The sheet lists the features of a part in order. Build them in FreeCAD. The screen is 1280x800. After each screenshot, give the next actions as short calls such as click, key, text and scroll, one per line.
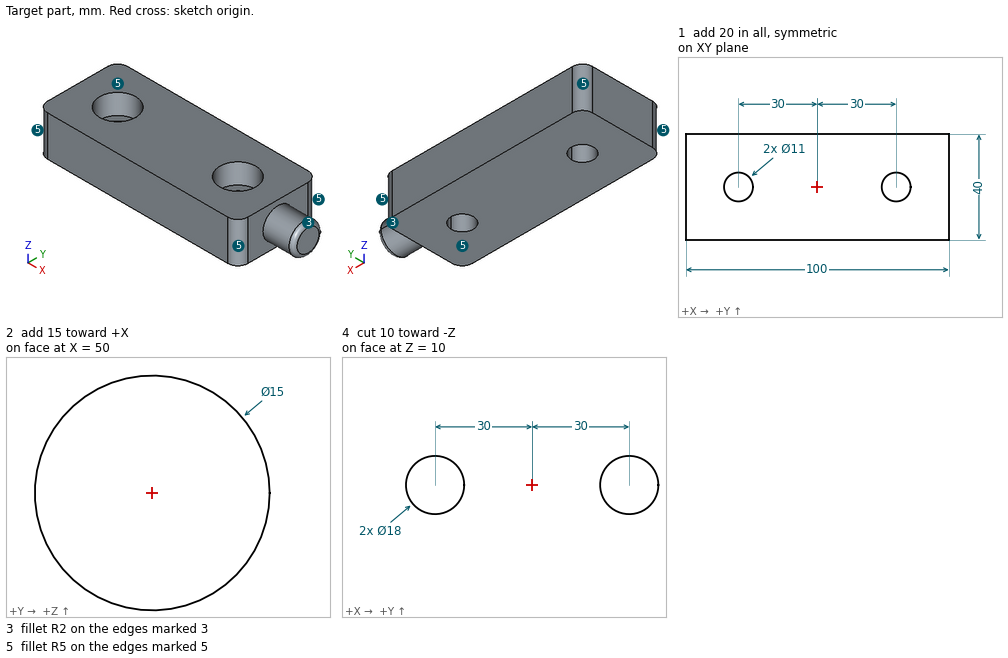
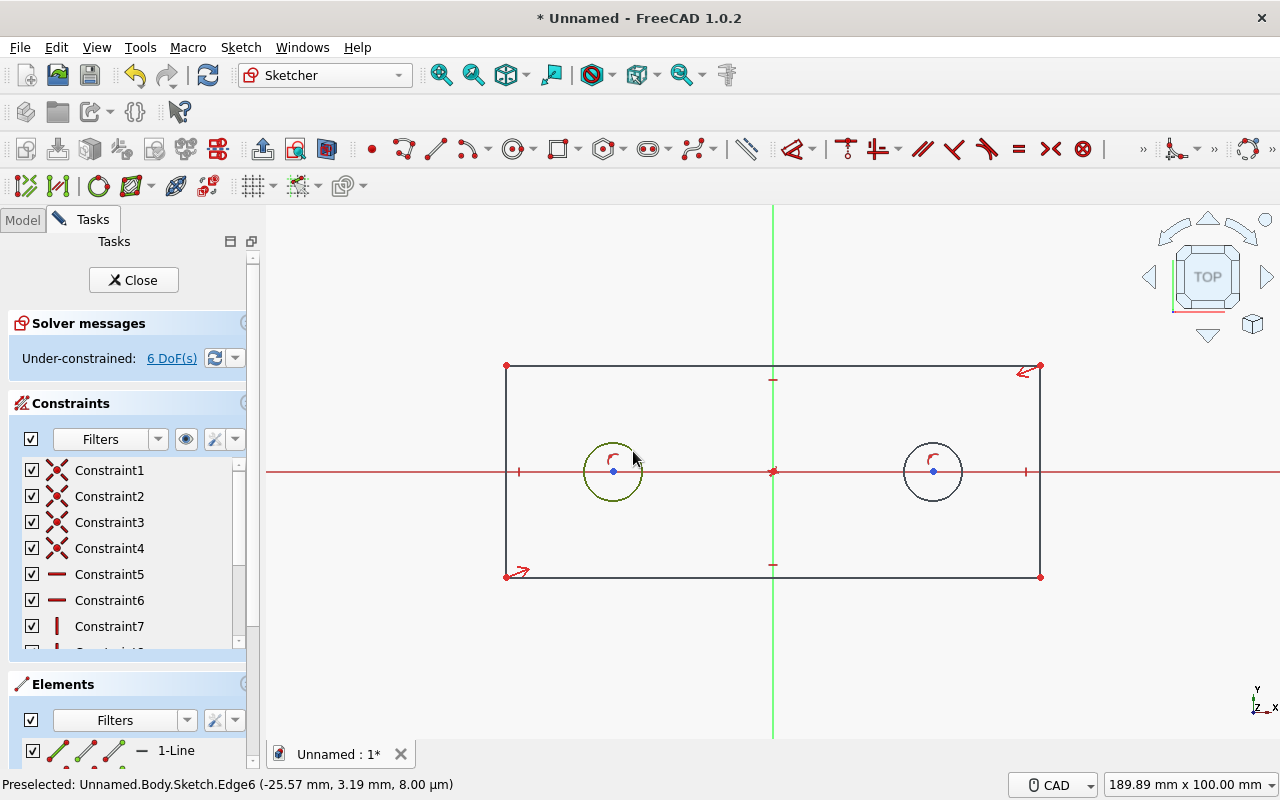
click(953, 451)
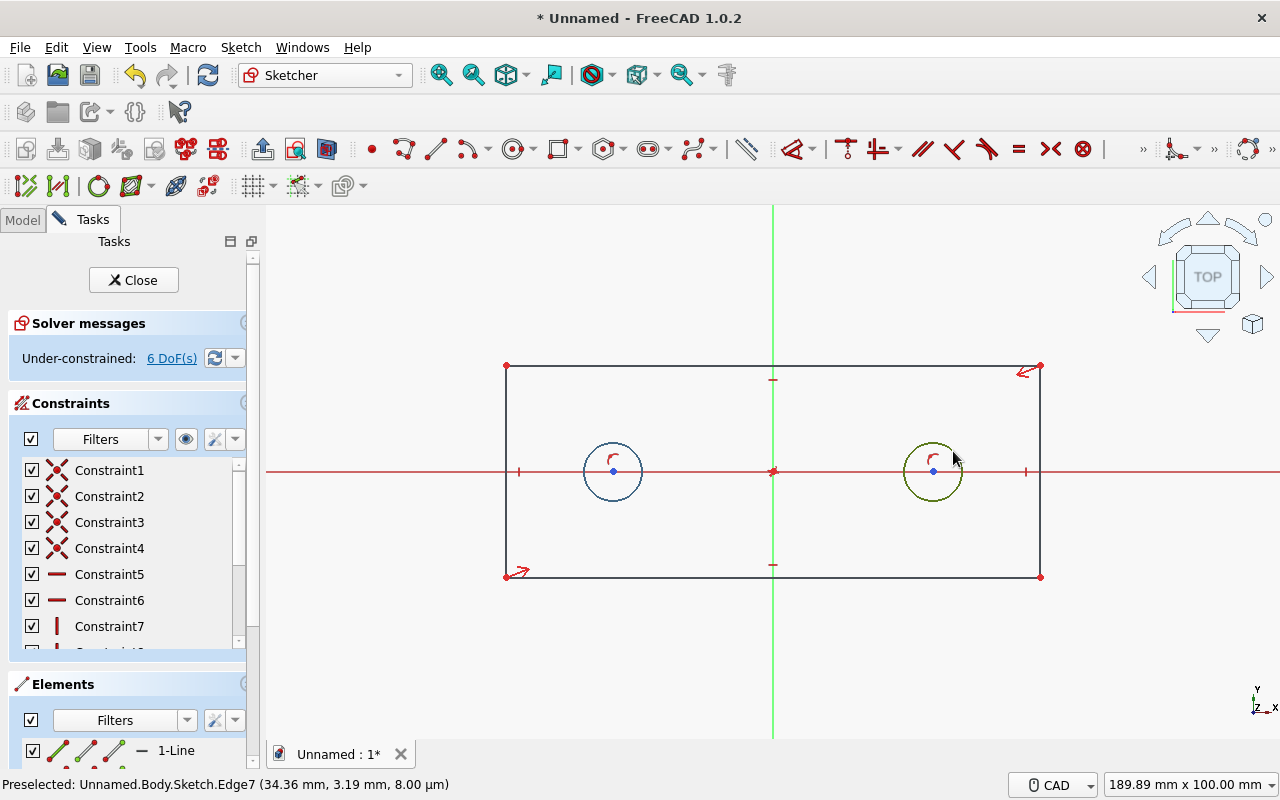
key(e)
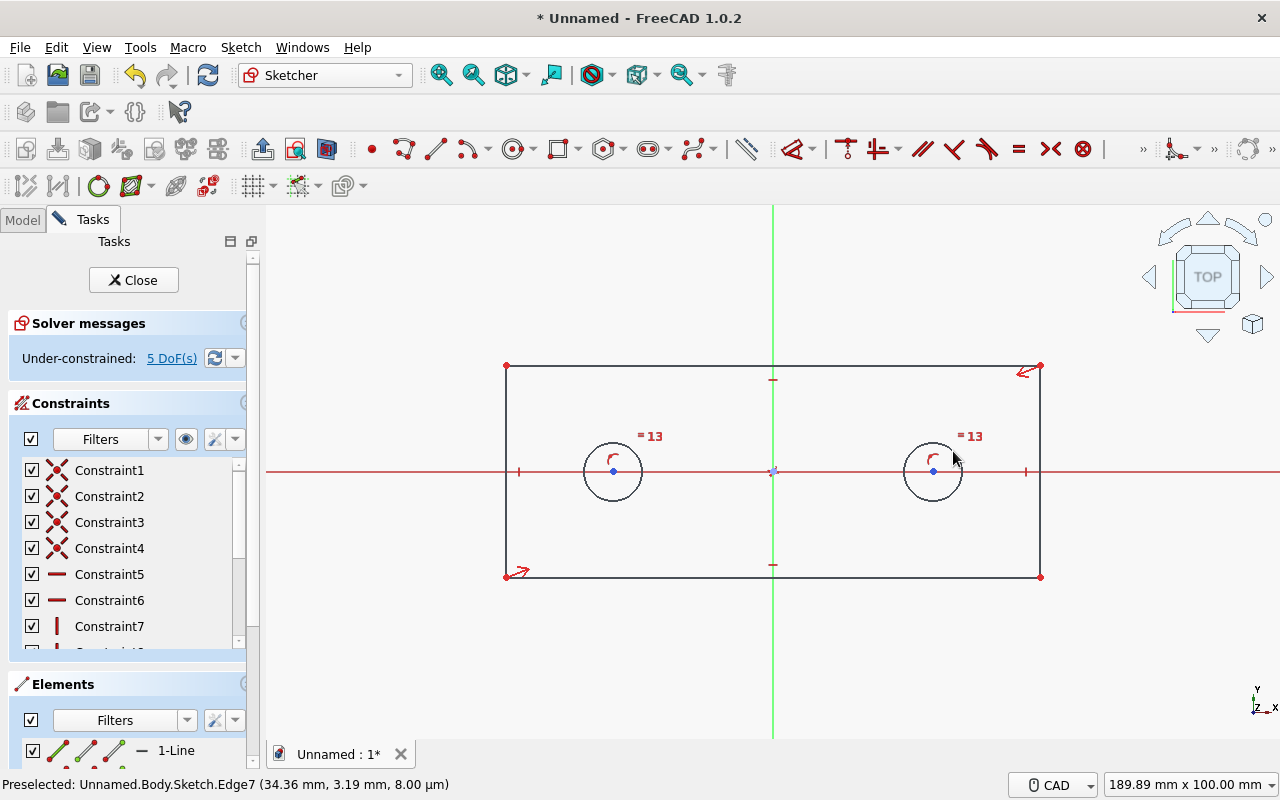
key(d)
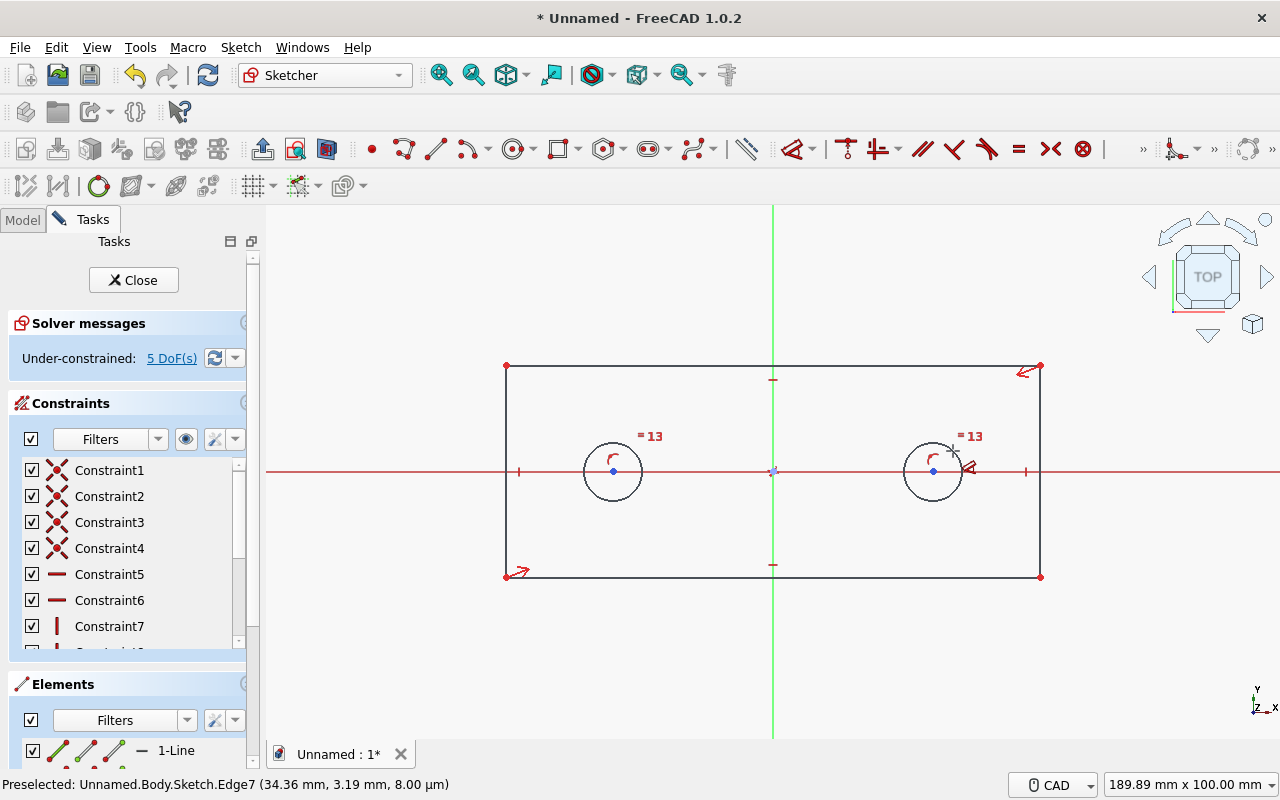
click(633, 451)
click(655, 428)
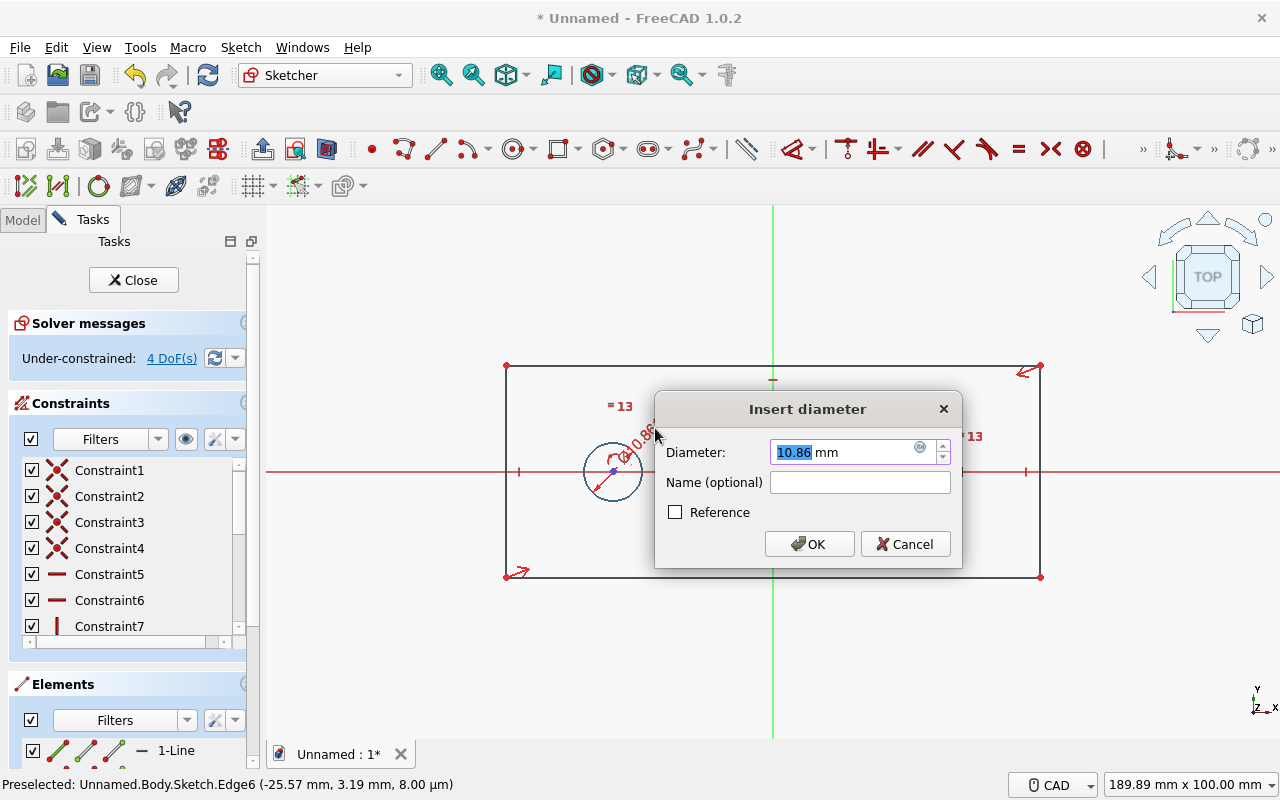
text(11)
key(Return)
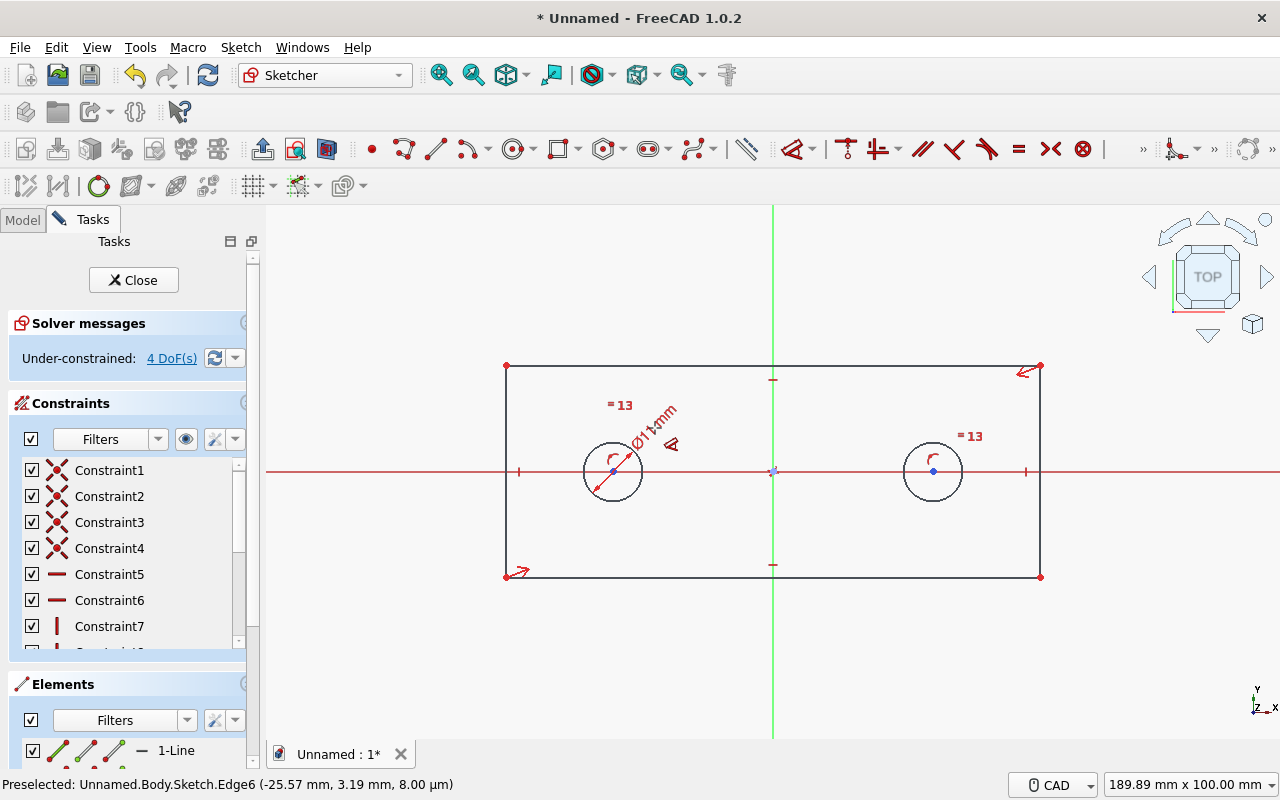
click(1040, 514)
click(1074, 423)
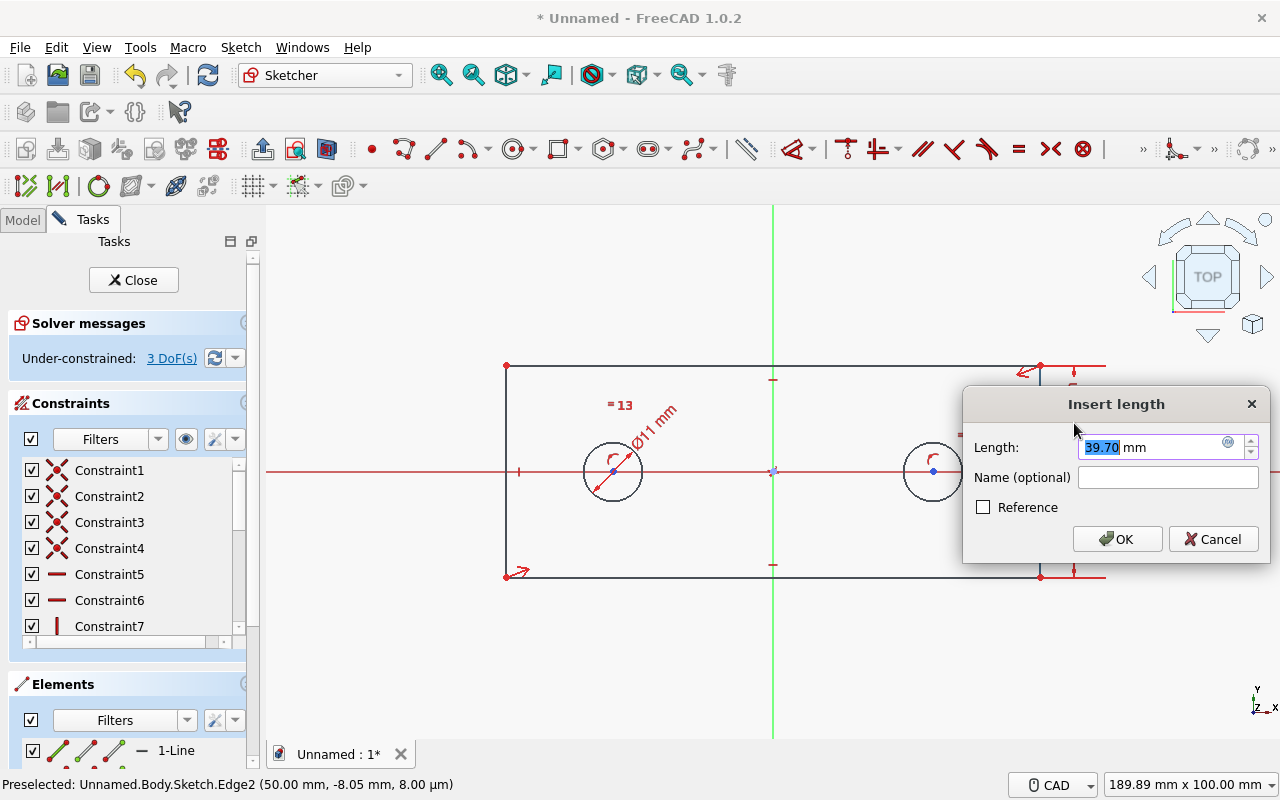
text(40)
key(Return)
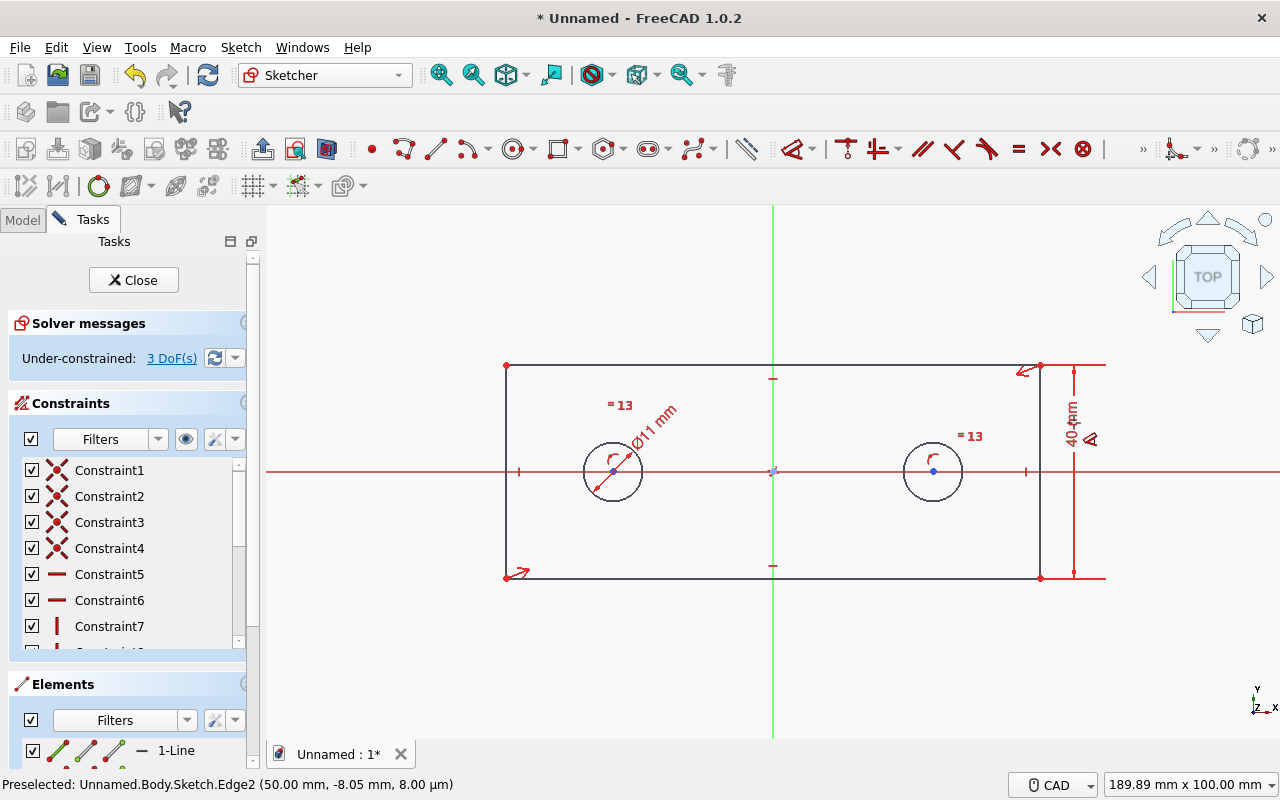
click(613, 472)
click(693, 506)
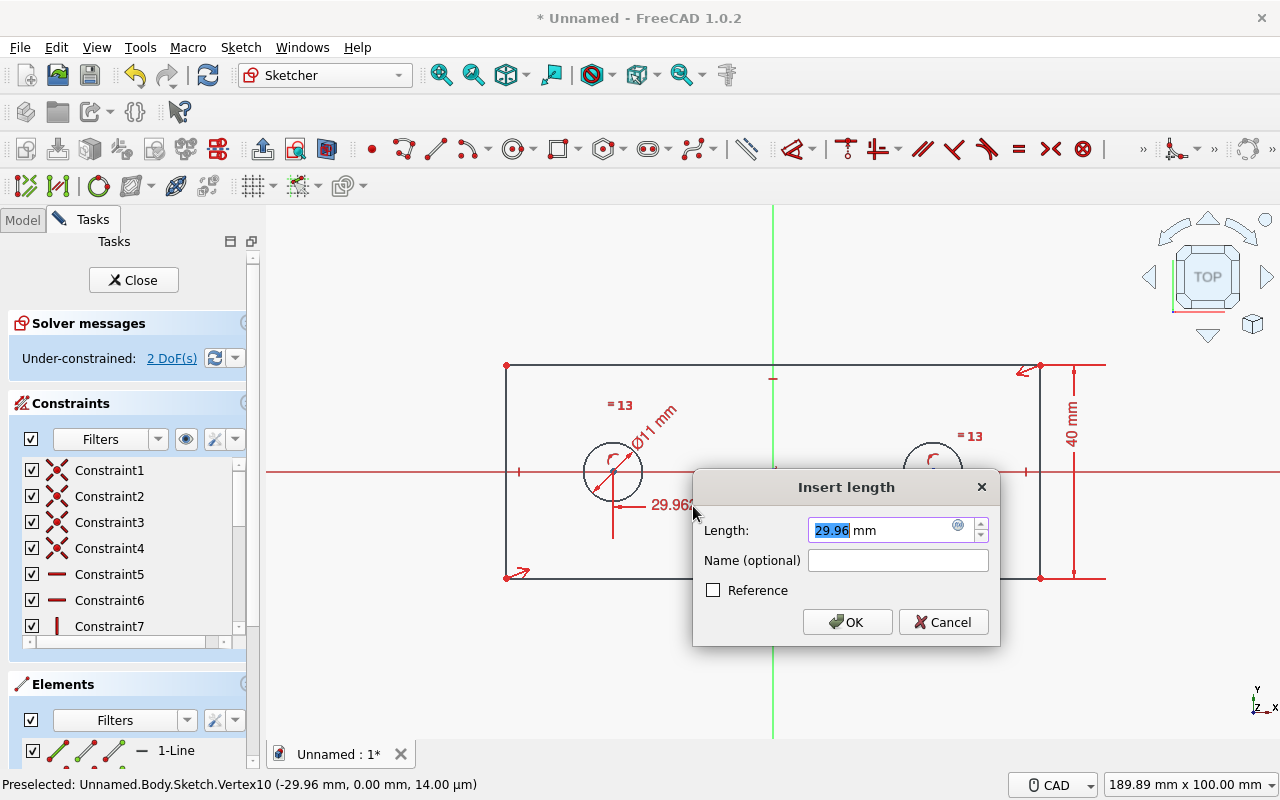
text(30)
key(Return)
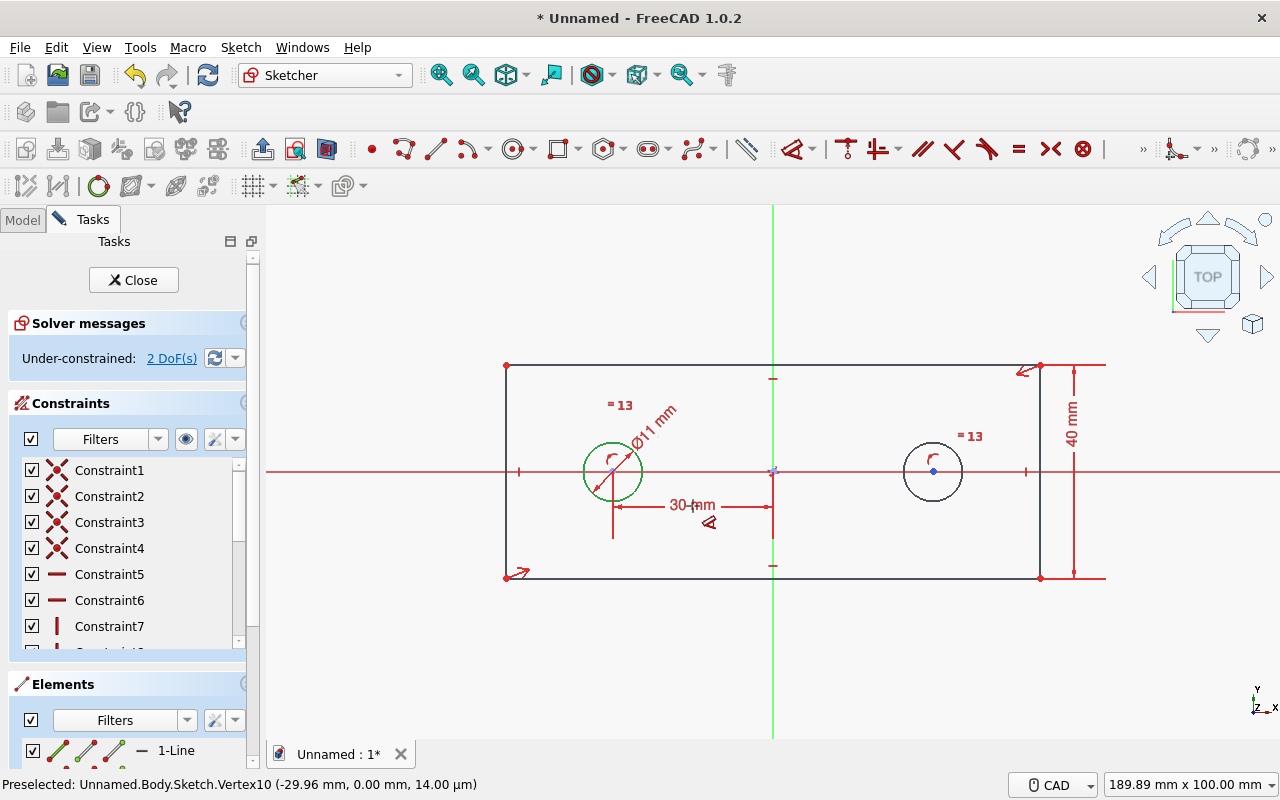
click(933, 472)
click(853, 506)